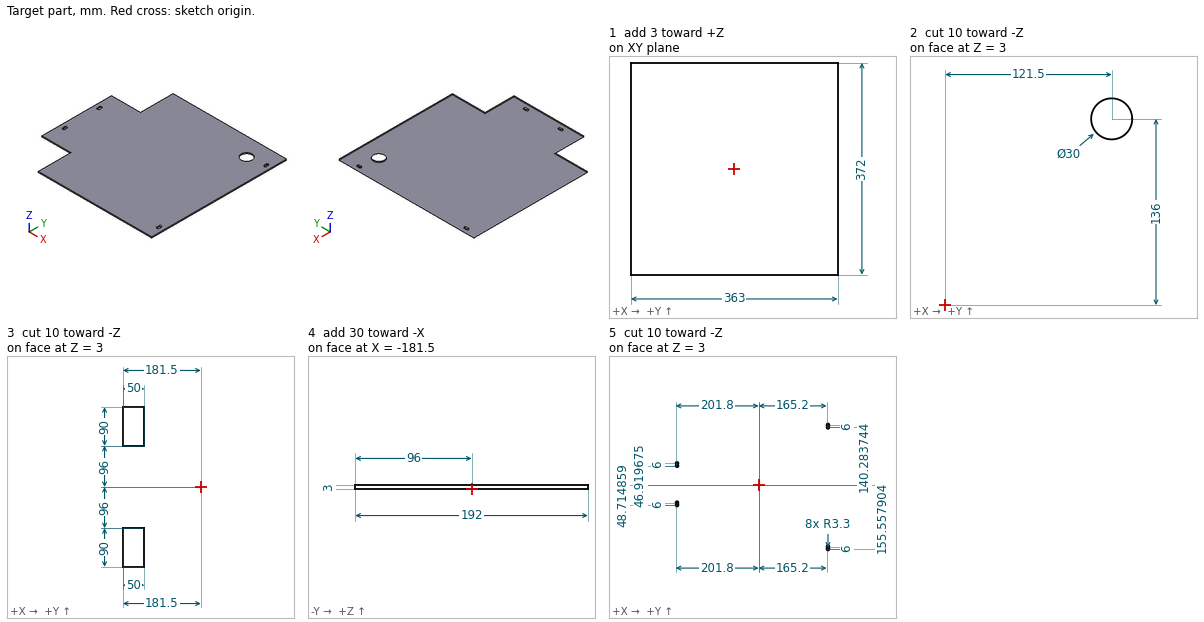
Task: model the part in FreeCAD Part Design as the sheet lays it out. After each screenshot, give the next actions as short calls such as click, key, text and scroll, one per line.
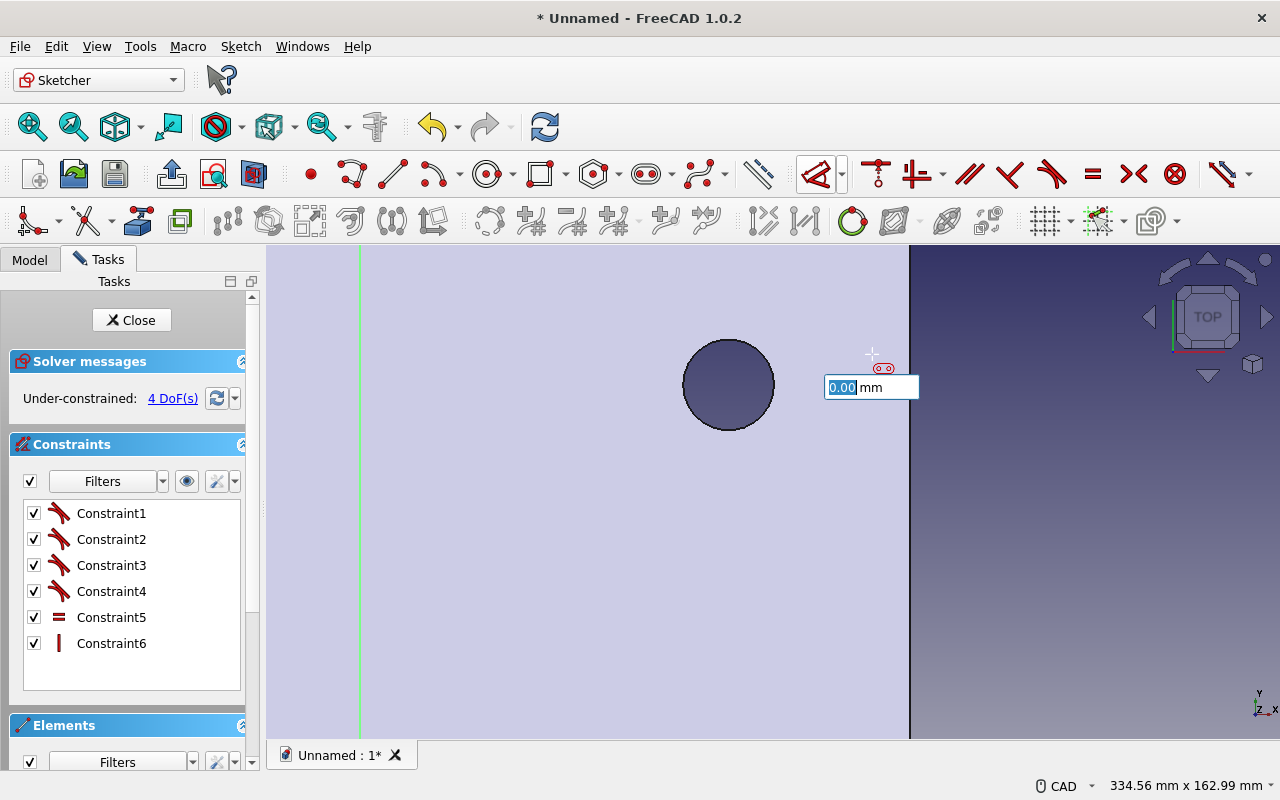
scroll(861, 363, up, 3)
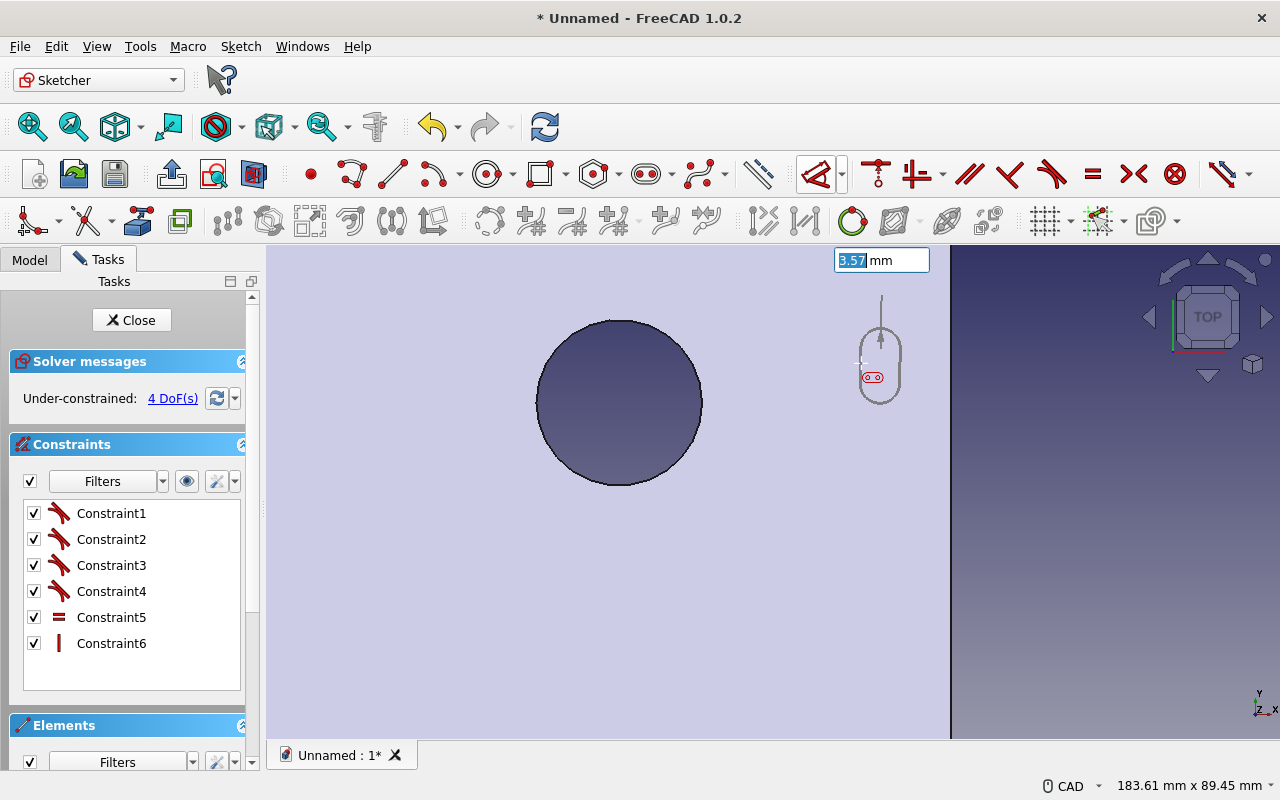
click(861, 363)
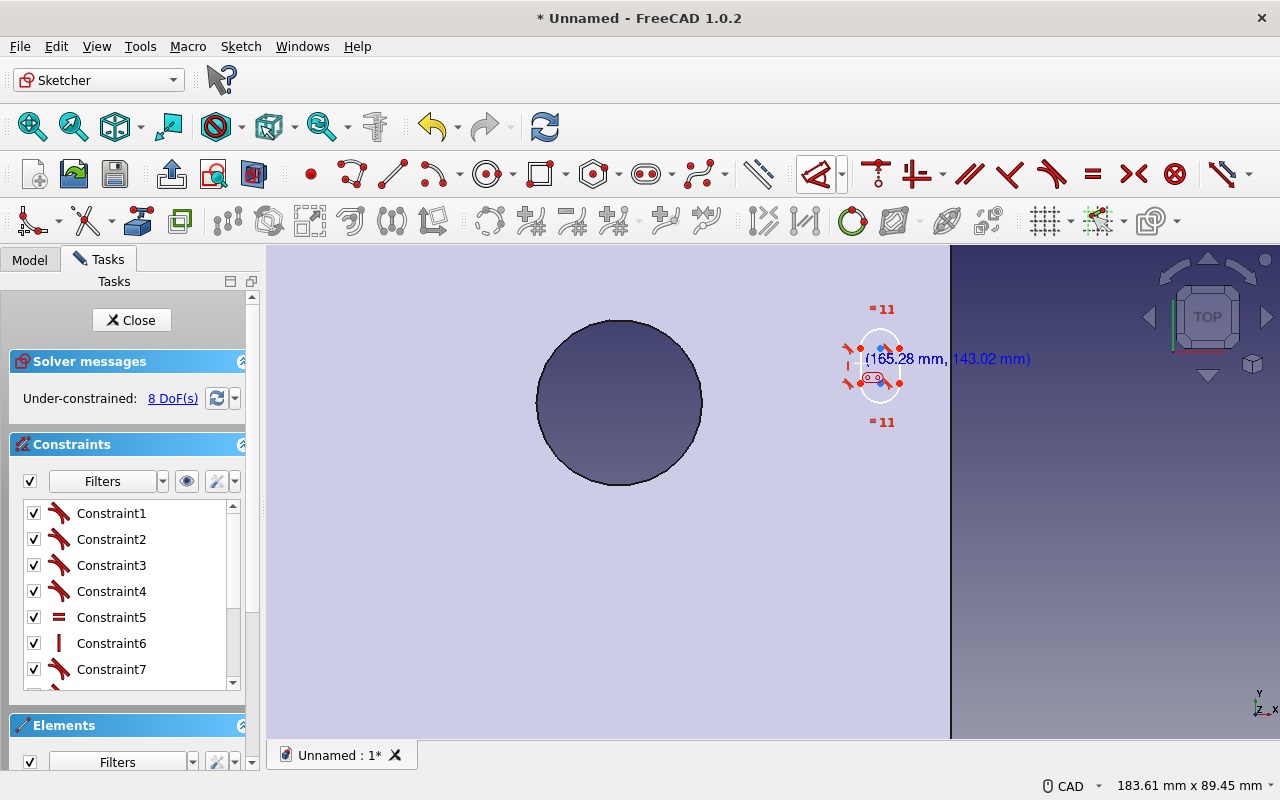
scroll(871, 356, down, 9)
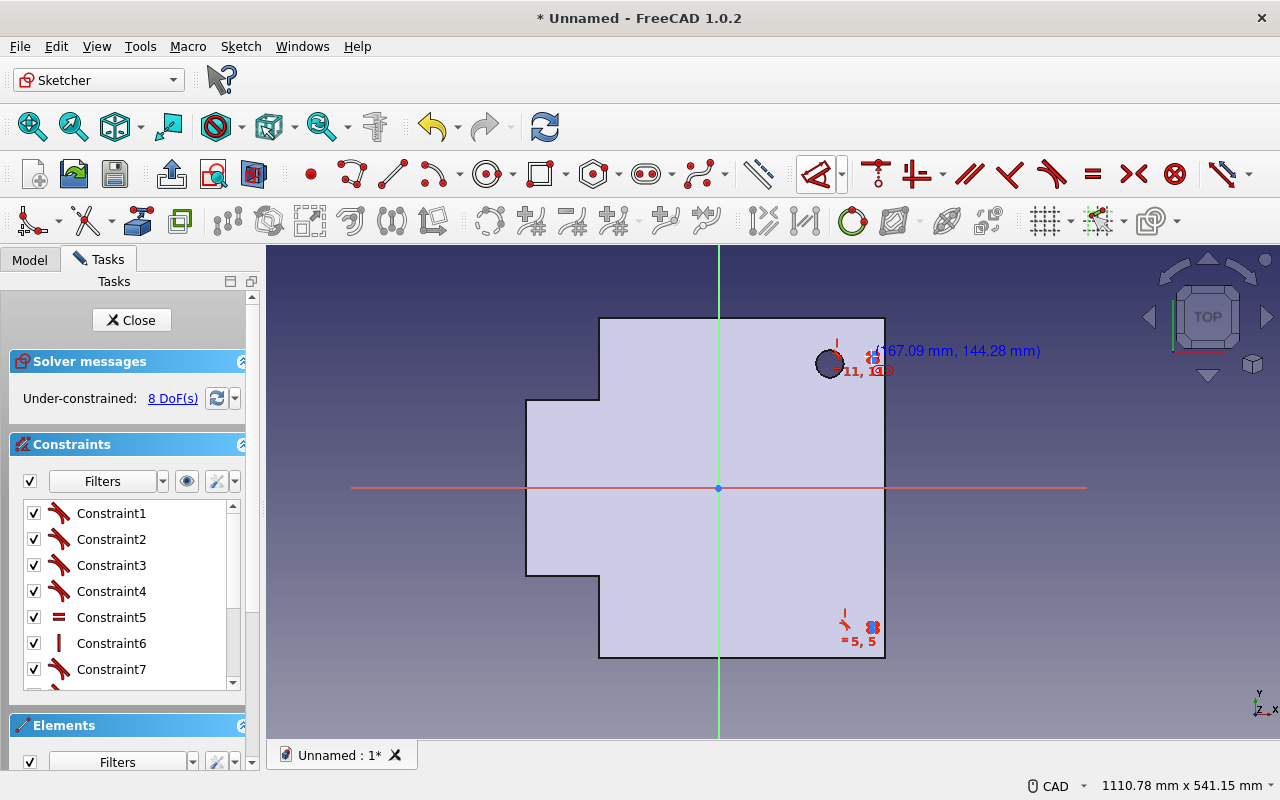
scroll(538, 445, up, 11)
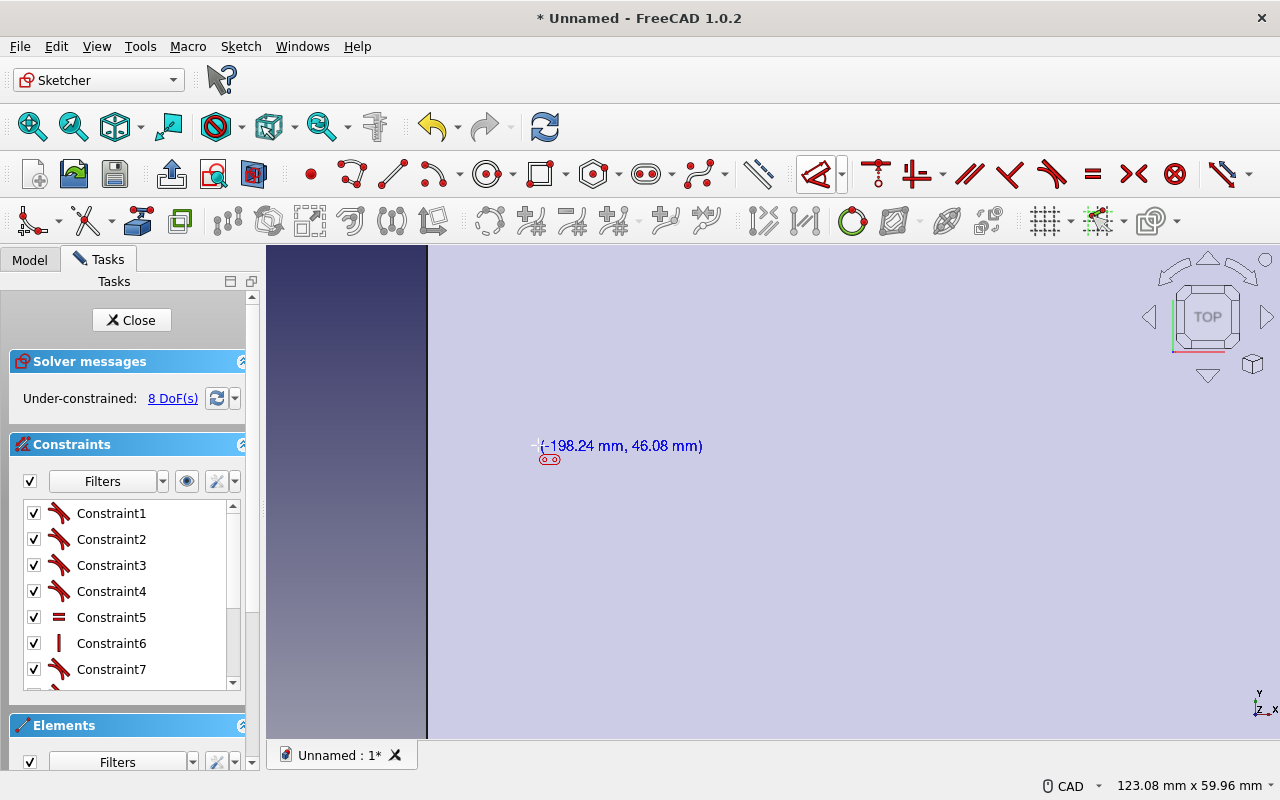
scroll(537, 445, down, 11)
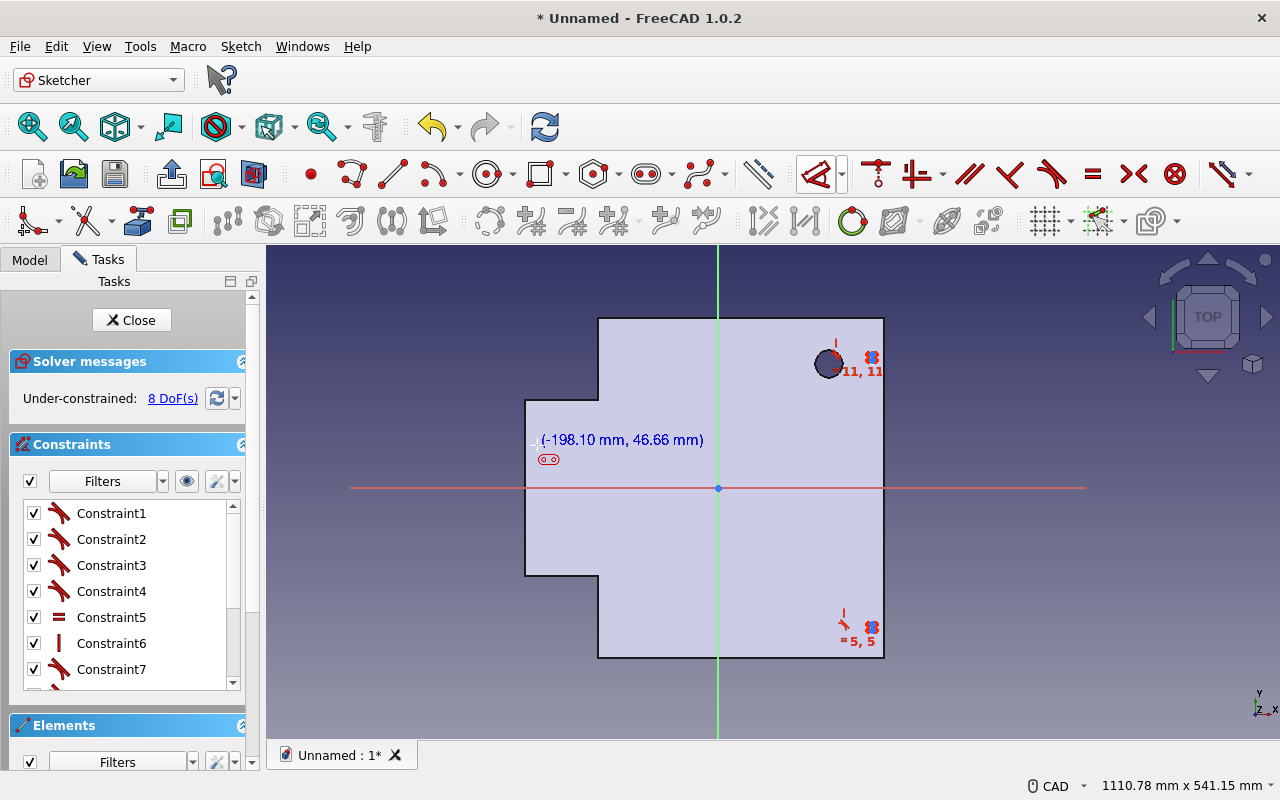
click(537, 445)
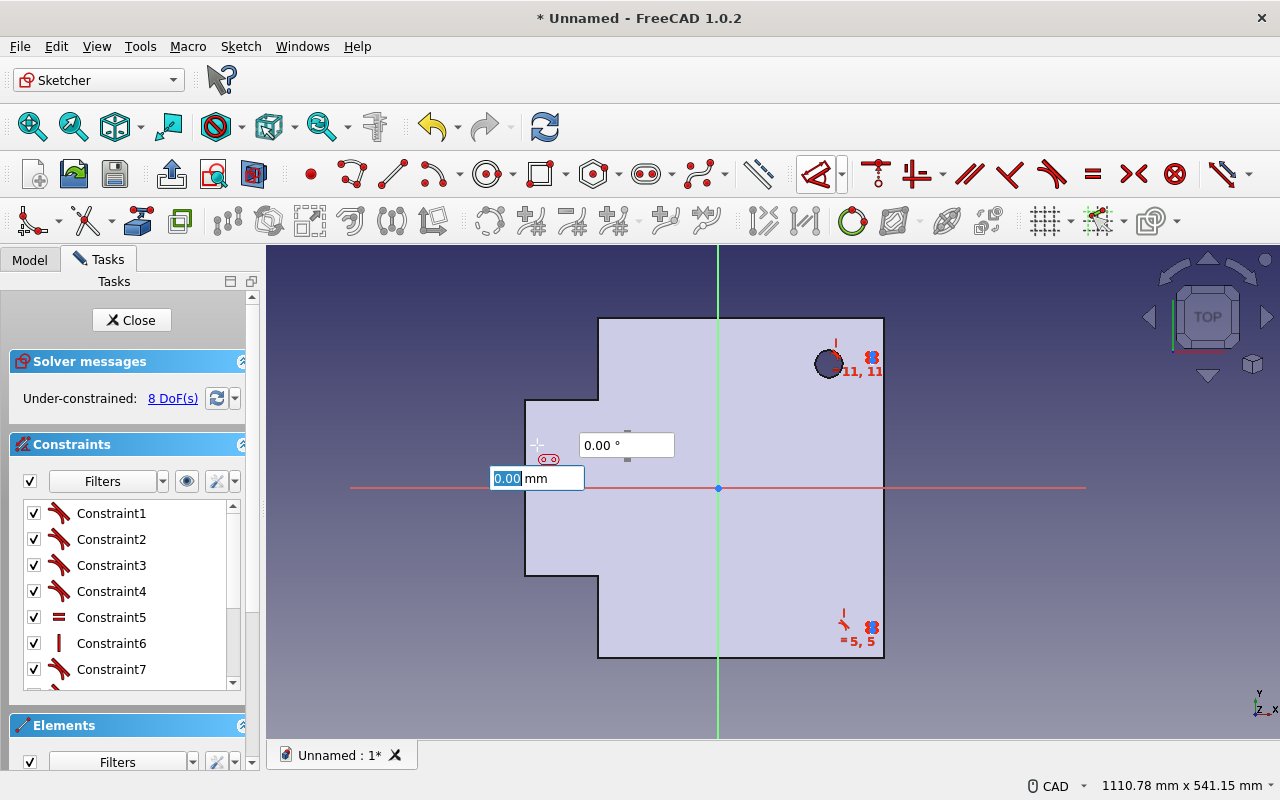
scroll(537, 440, up, 6)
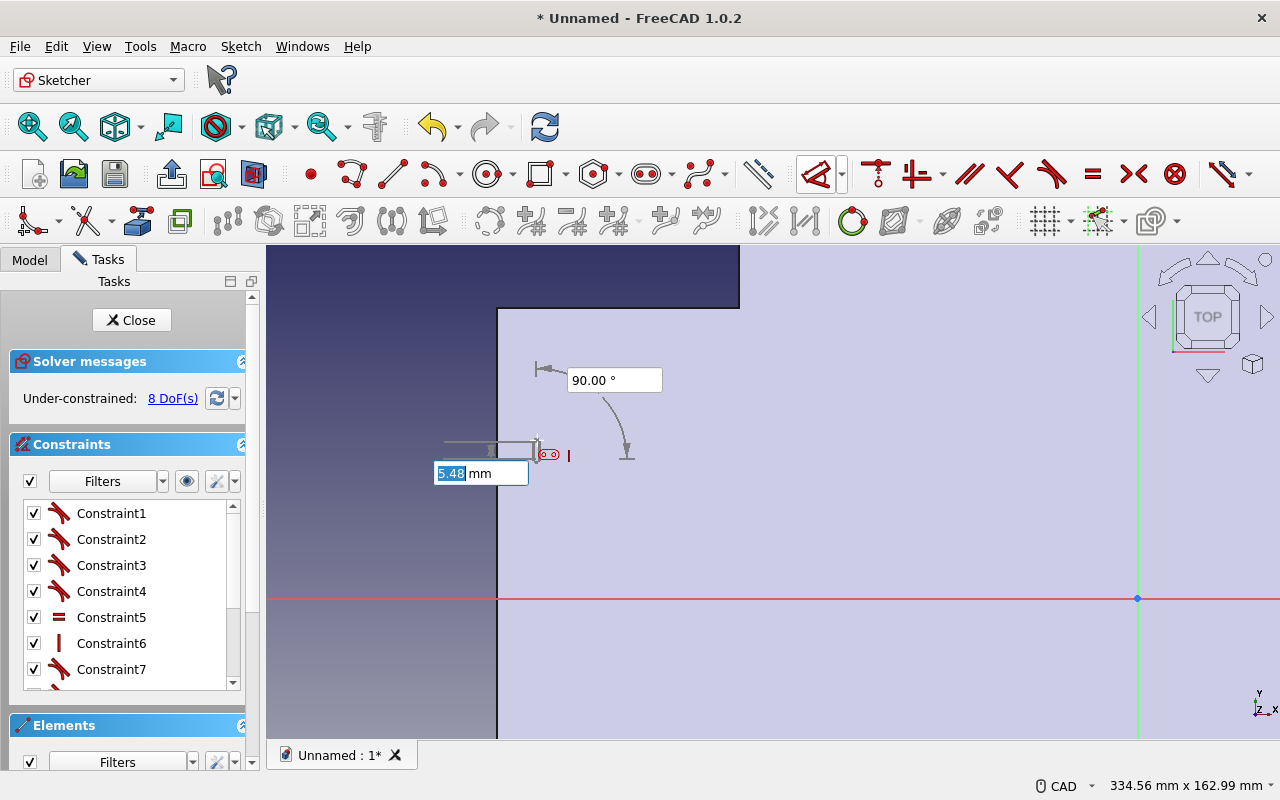
click(536, 438)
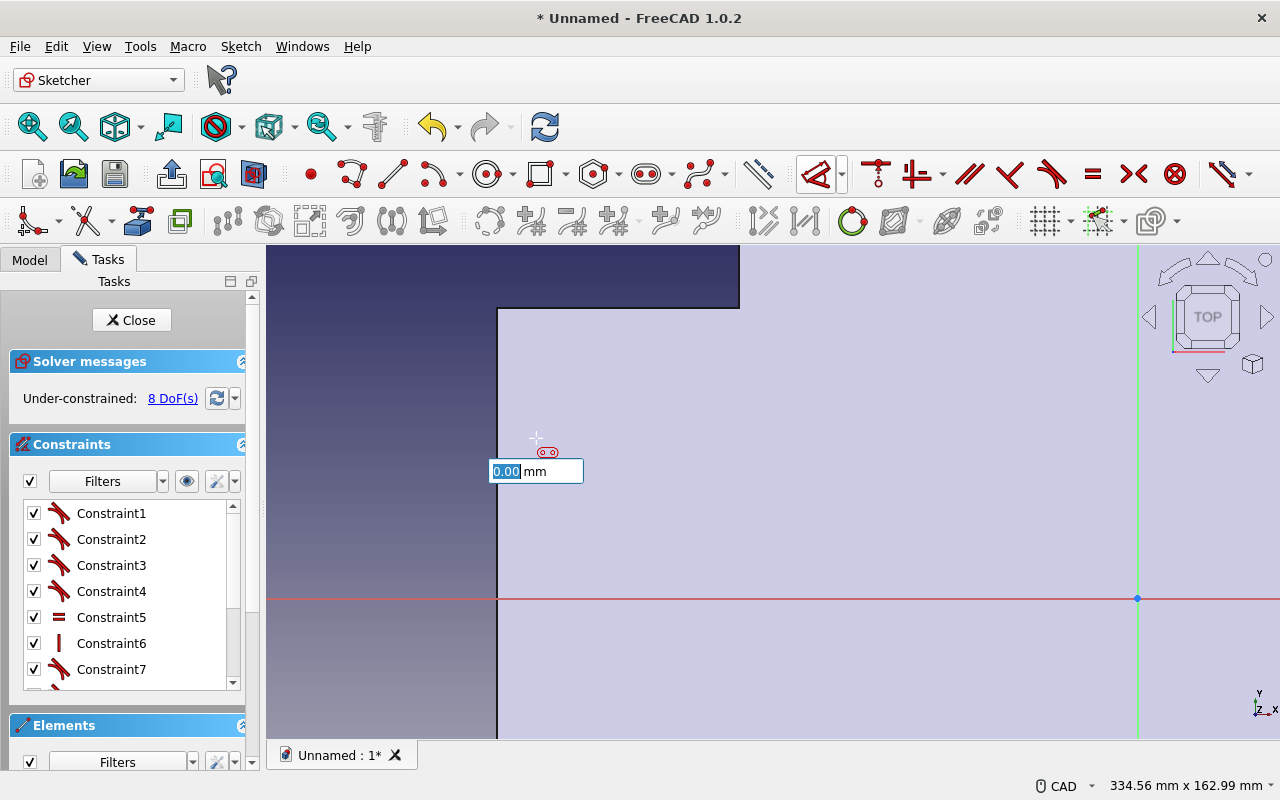
scroll(546, 447, up, 3)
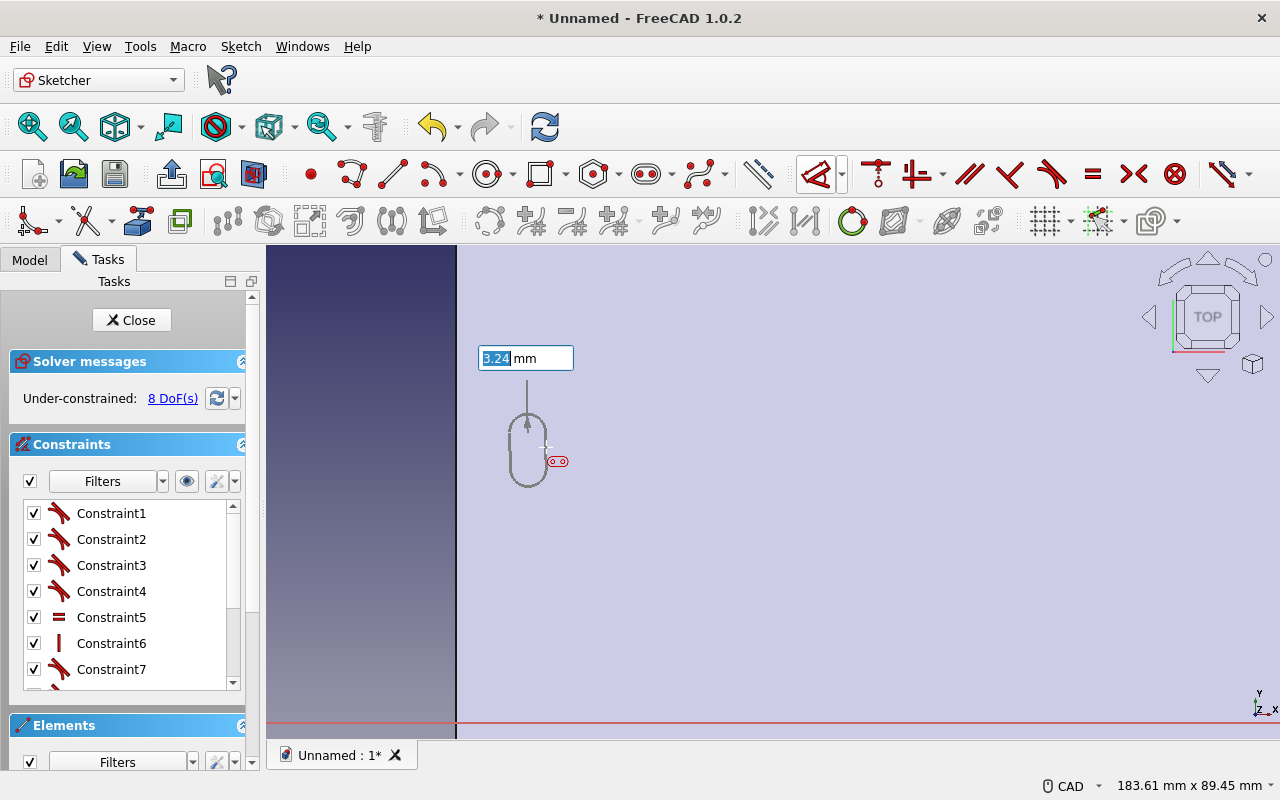
click(546, 447)